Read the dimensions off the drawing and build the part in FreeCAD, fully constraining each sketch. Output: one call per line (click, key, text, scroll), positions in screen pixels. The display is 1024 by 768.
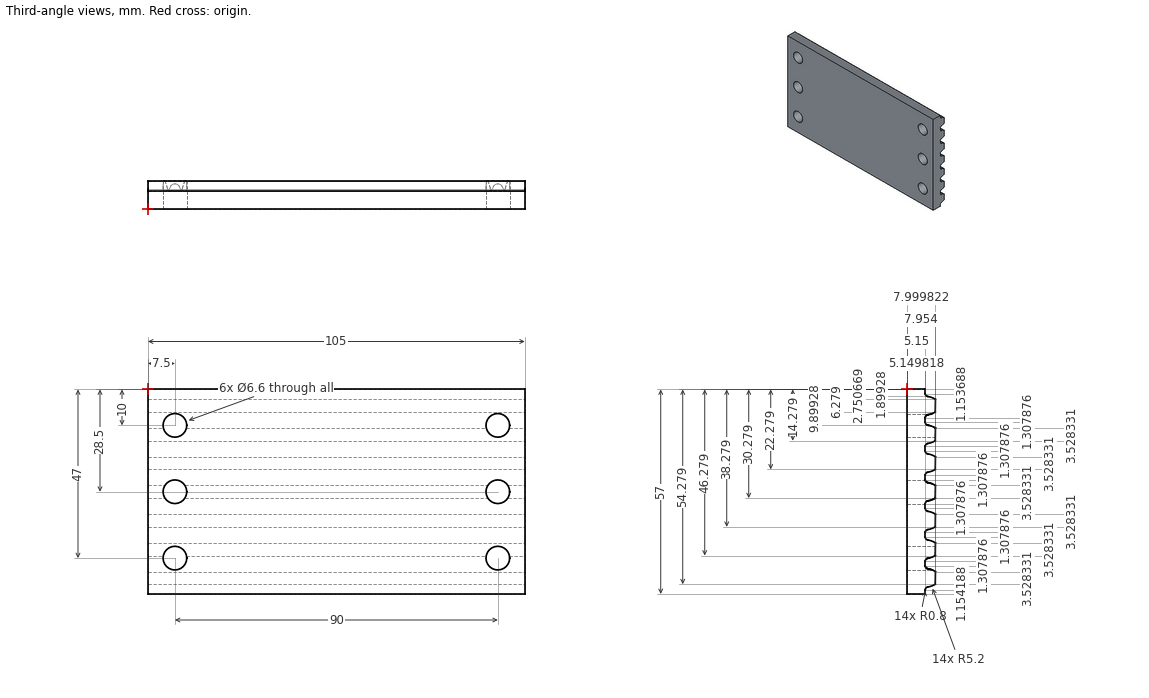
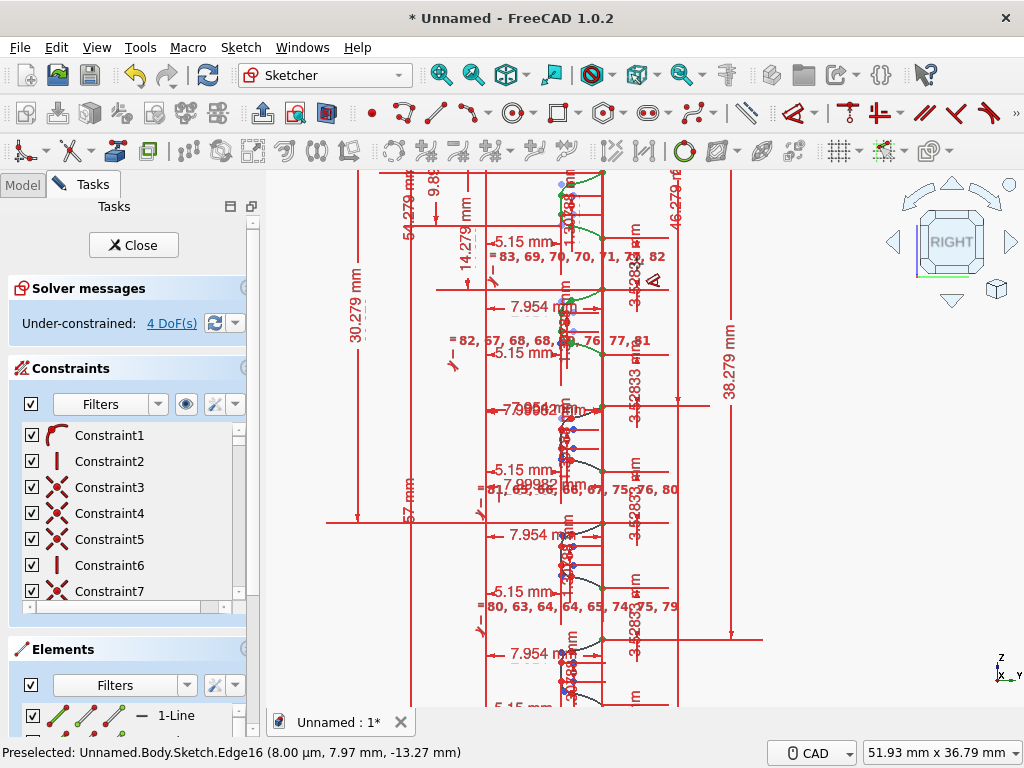
scroll(603, 391, down, 4)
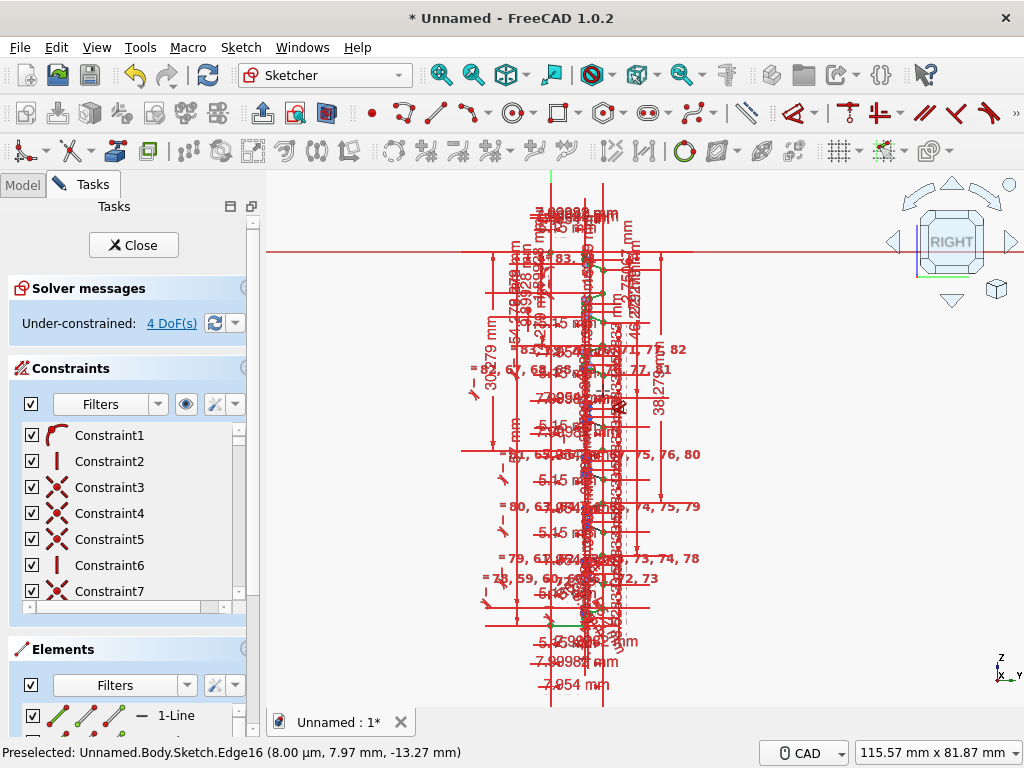
scroll(583, 613, up, 4)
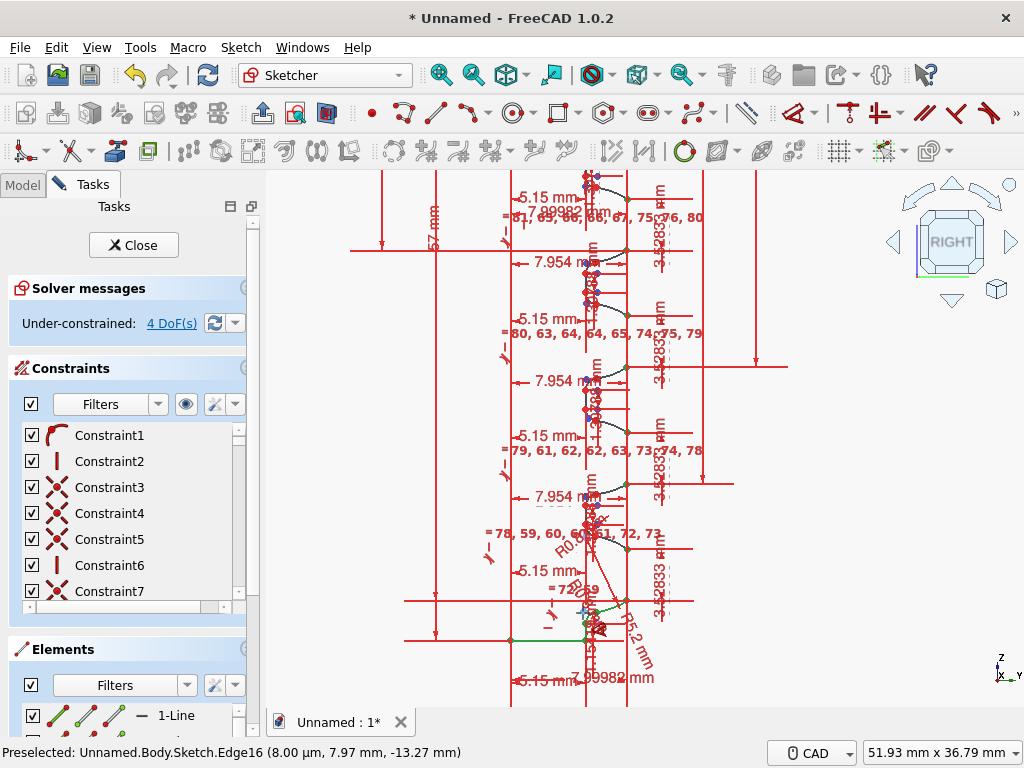
click(583, 611)
click(547, 669)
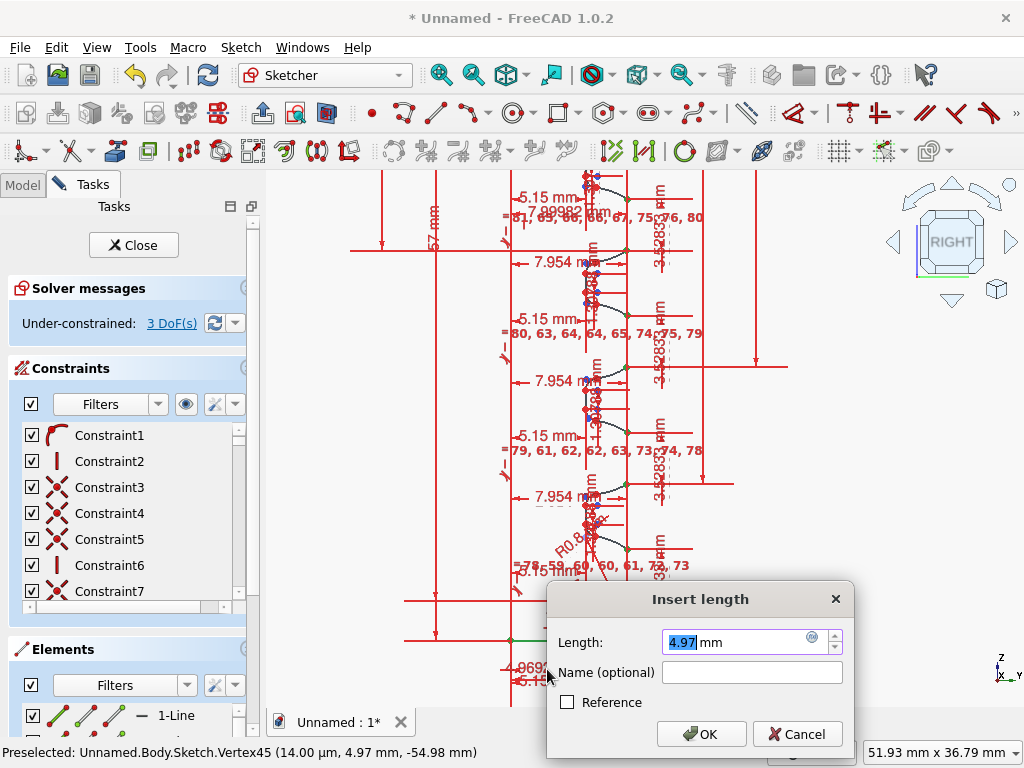
text(5.149818)
key(Return)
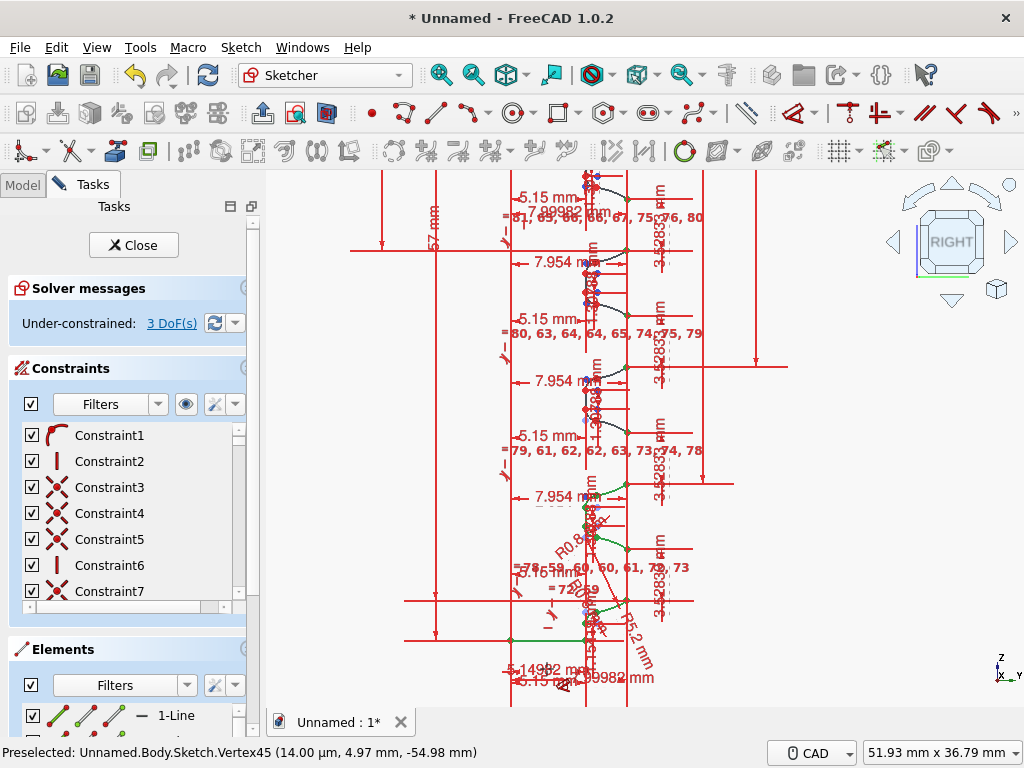
click(586, 496)
click(531, 530)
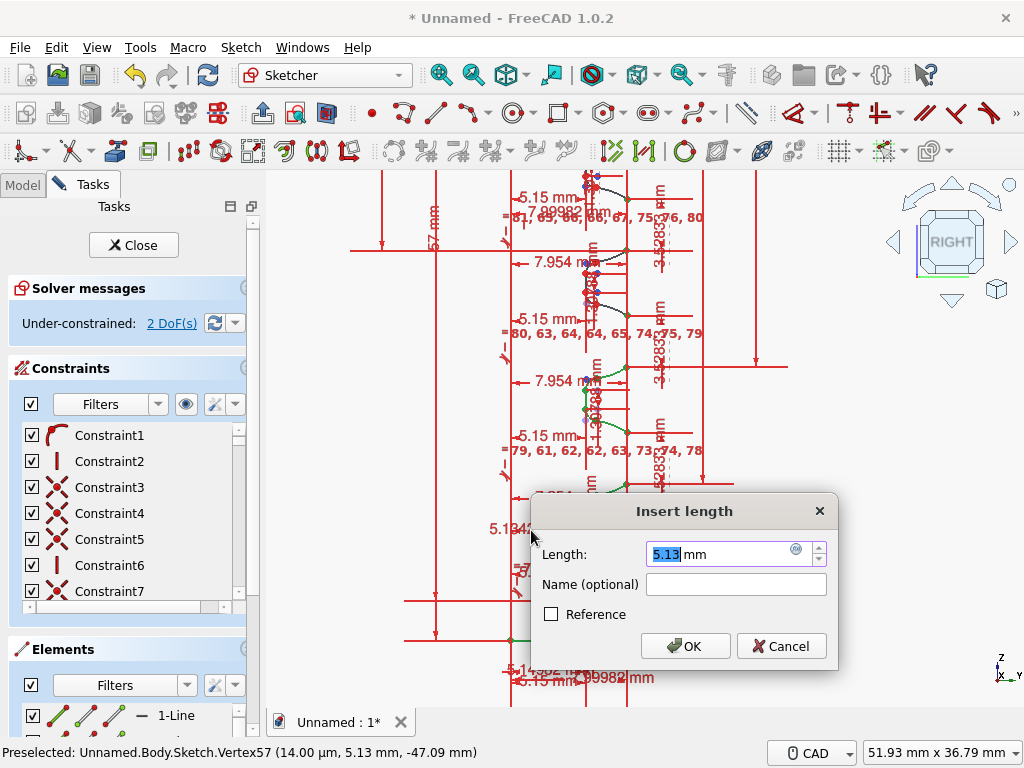
text(5.149818)
key(Return)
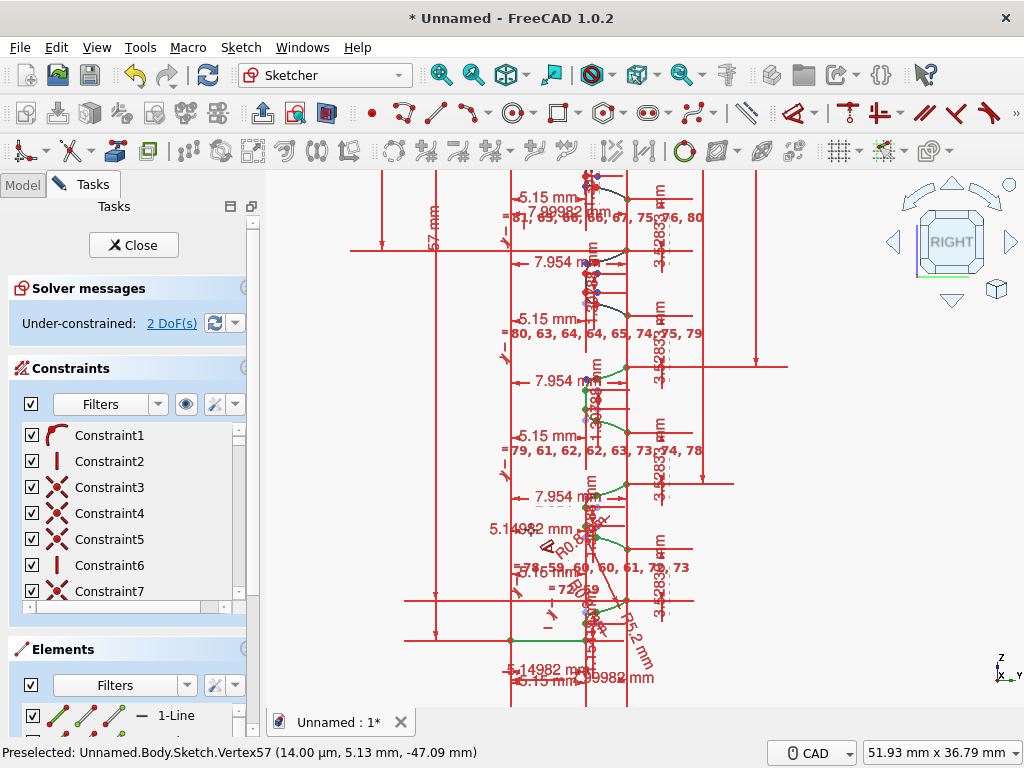
scroll(586, 380, up, 2)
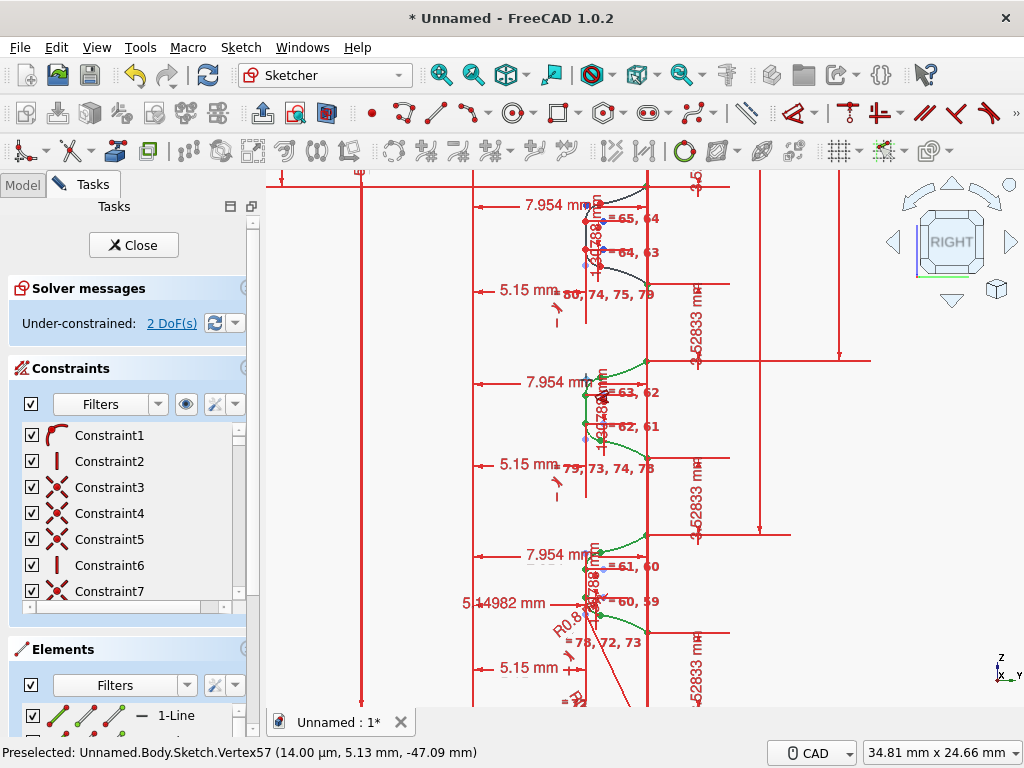
click(586, 379)
click(530, 413)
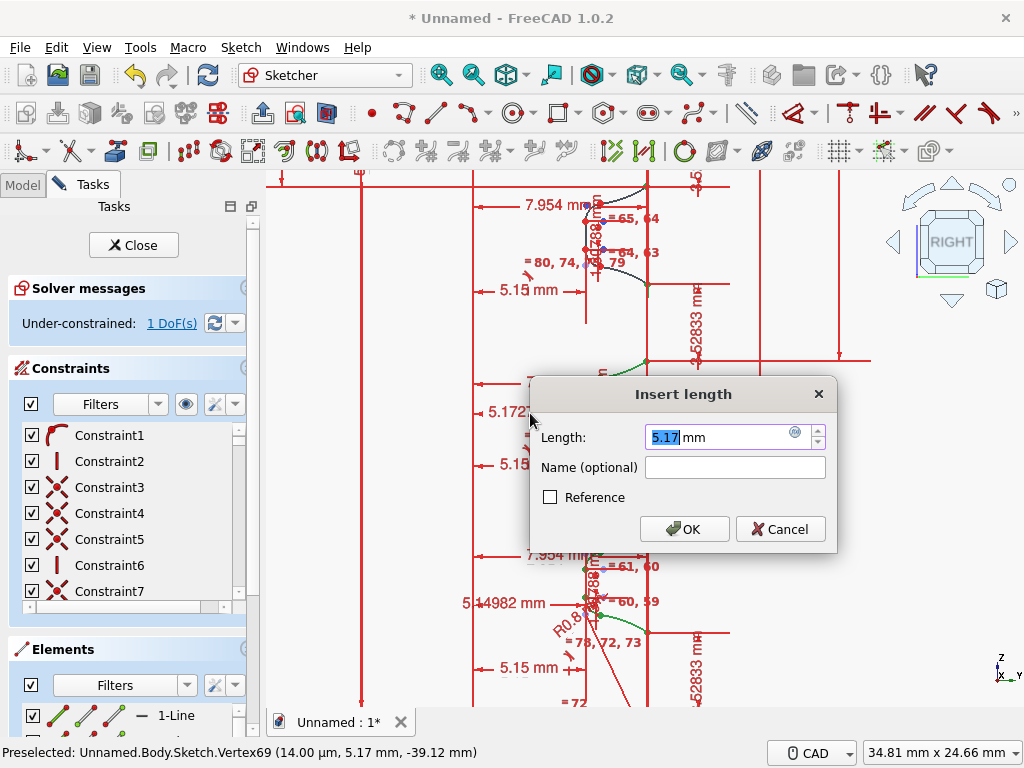
text(5.149818)
key(Return)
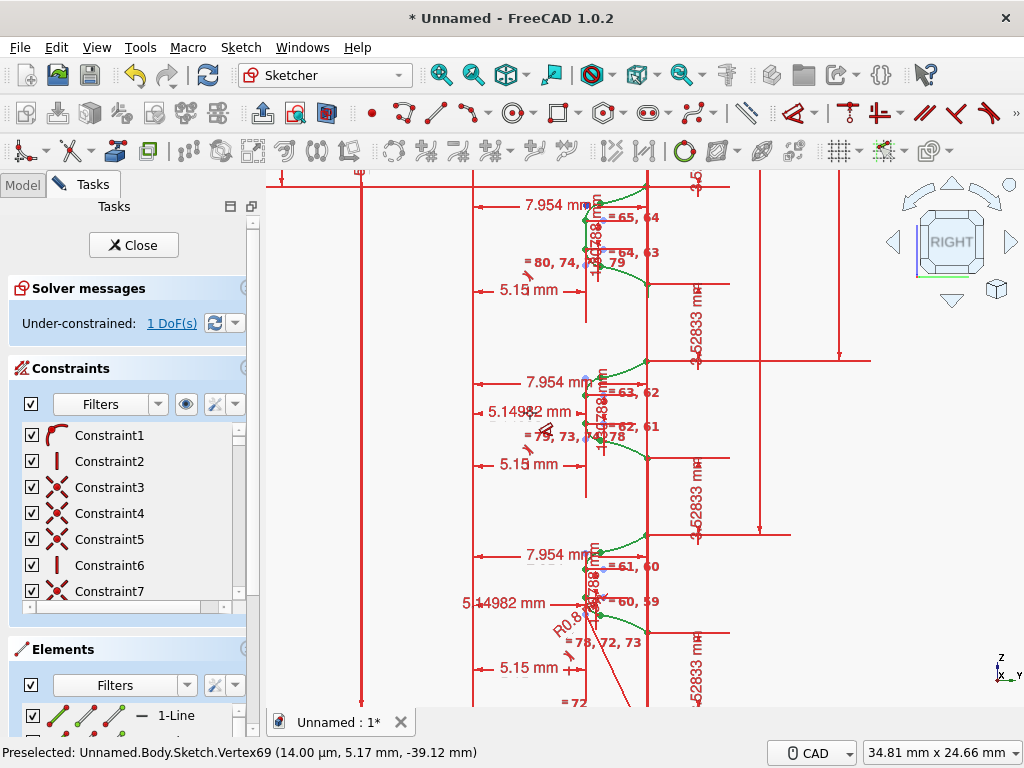
click(587, 205)
click(504, 239)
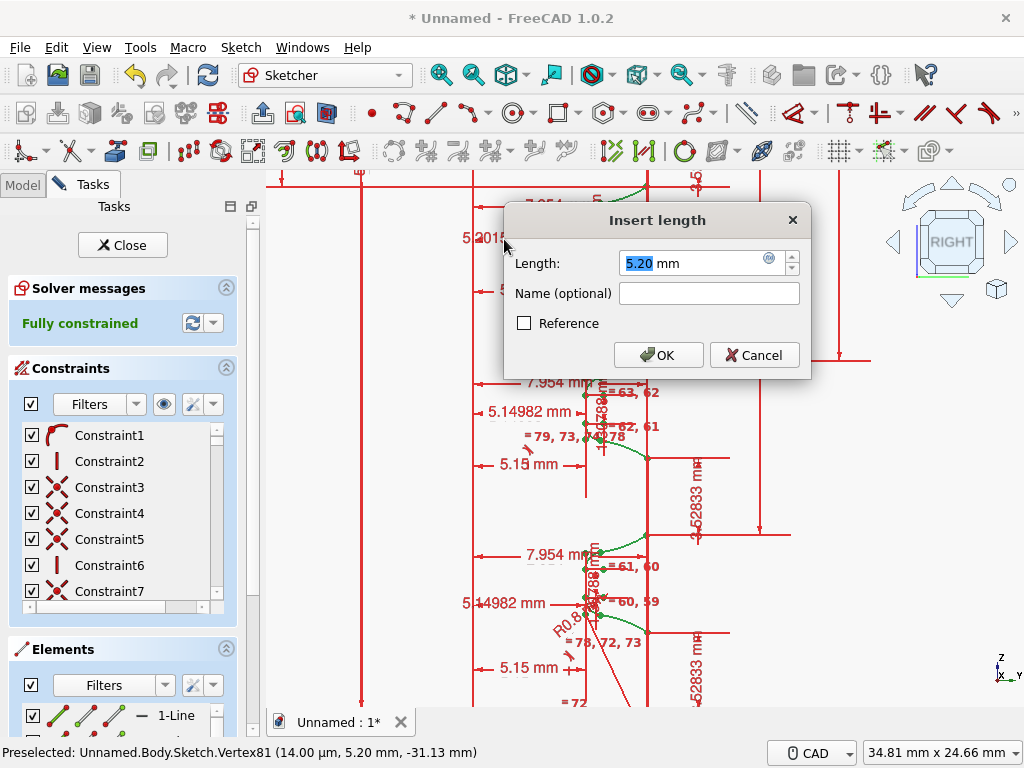
text(5.149818)
key(Return)
key(Escape)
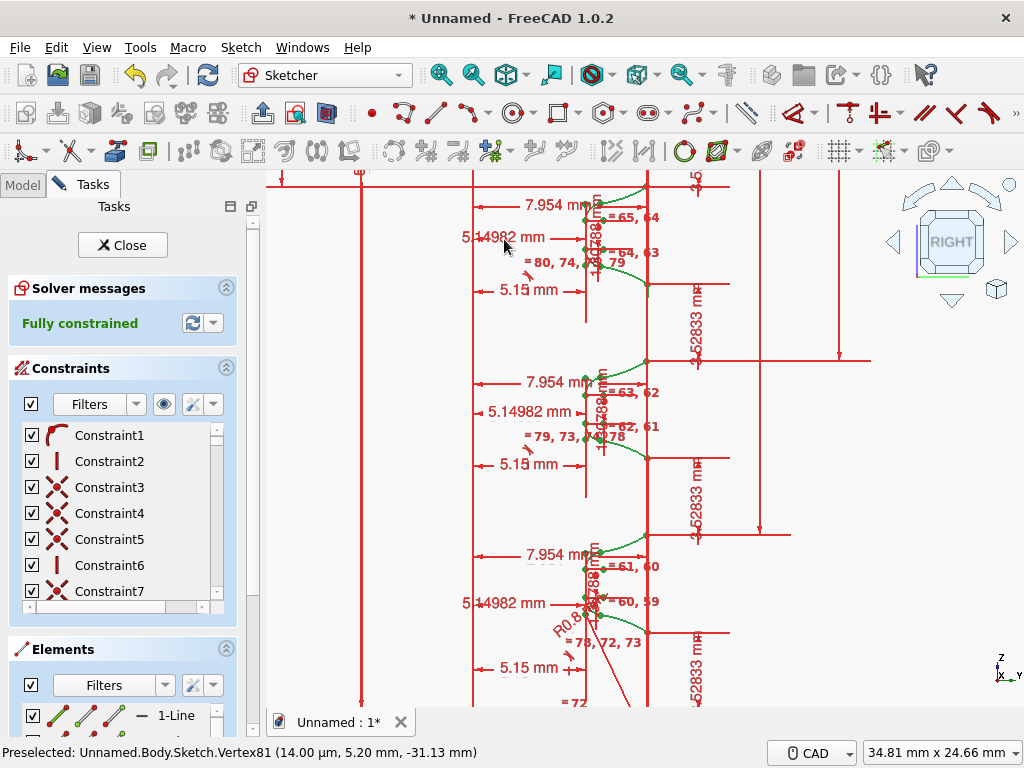
click(123, 245)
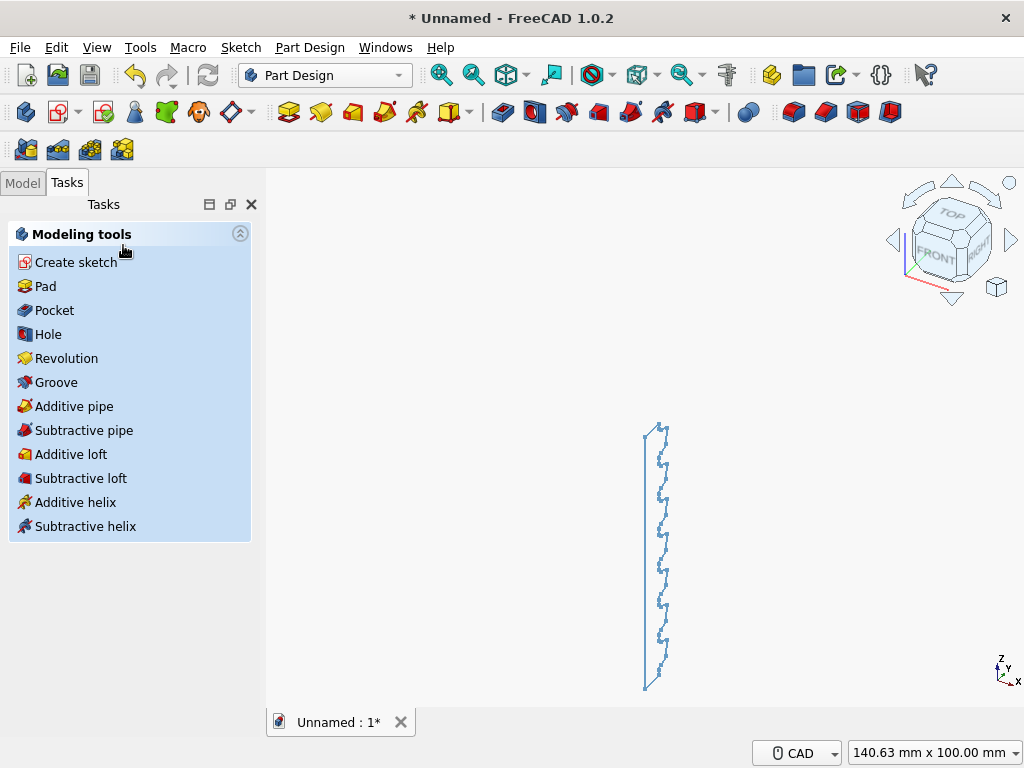
click(290, 112)